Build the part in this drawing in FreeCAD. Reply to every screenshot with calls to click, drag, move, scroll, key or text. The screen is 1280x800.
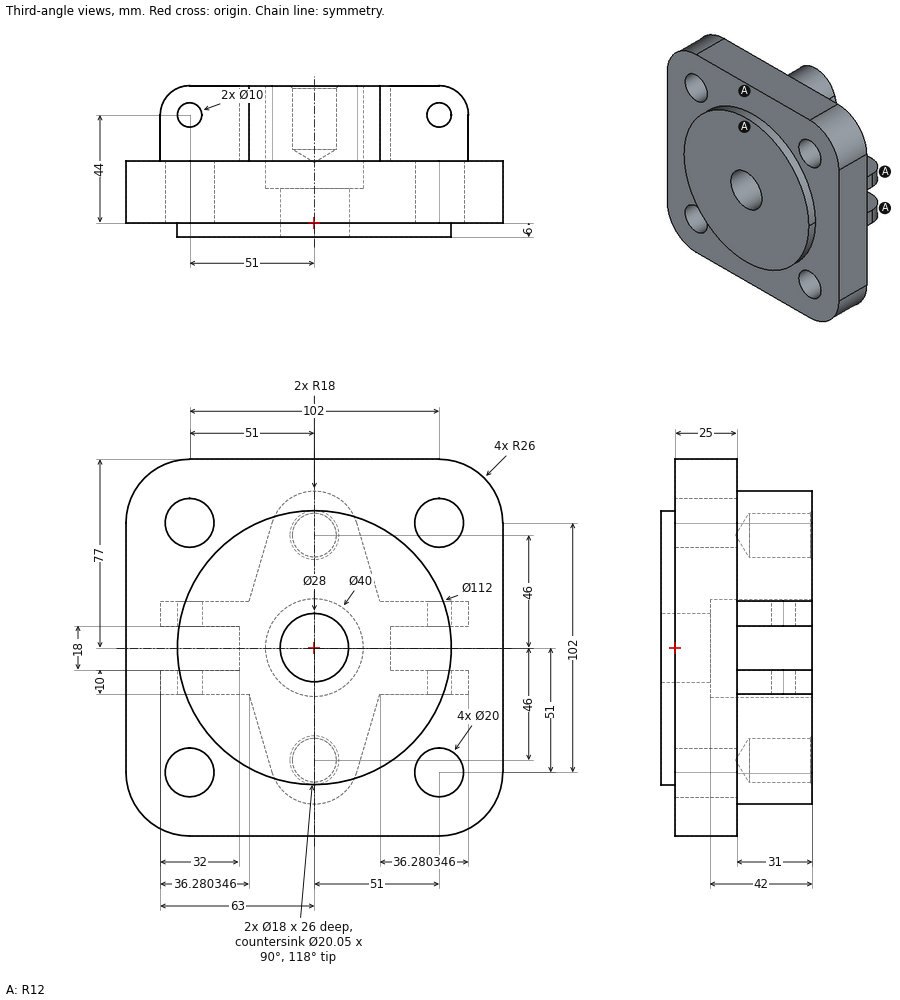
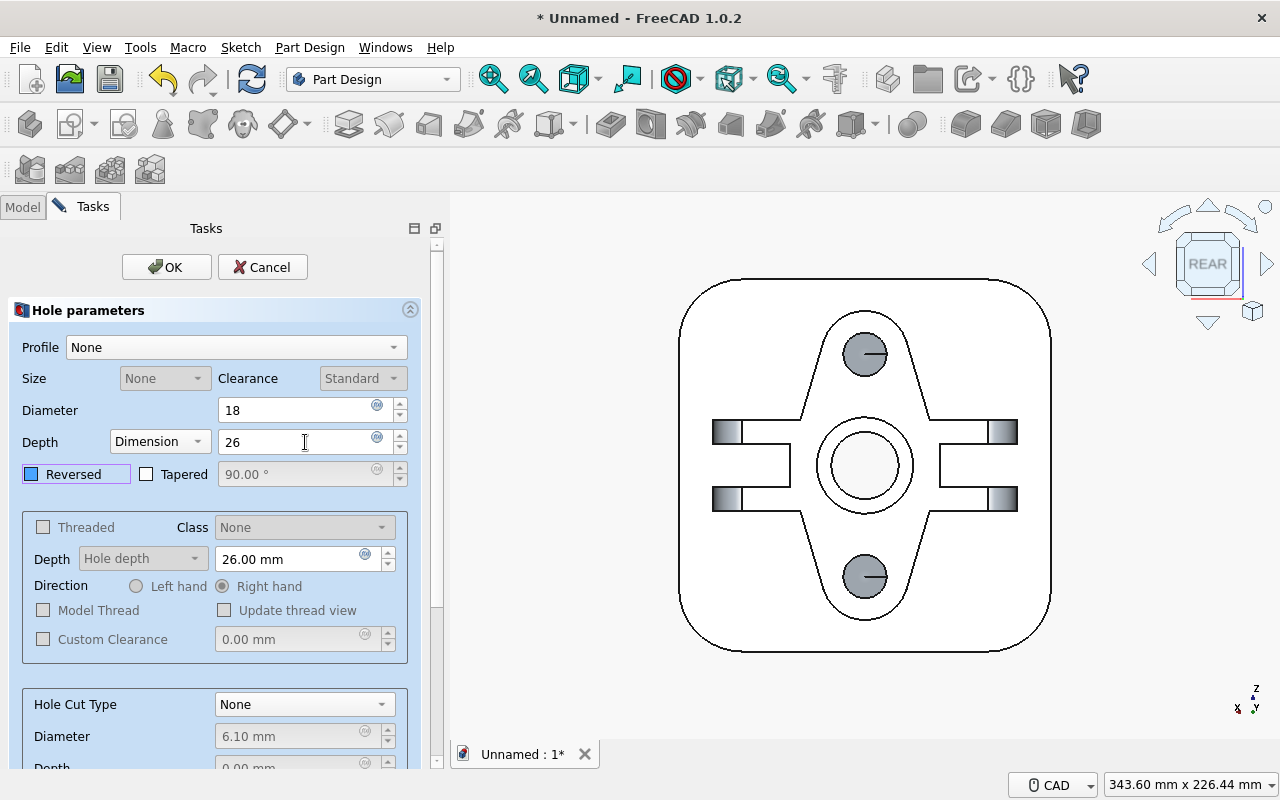
click(306, 704)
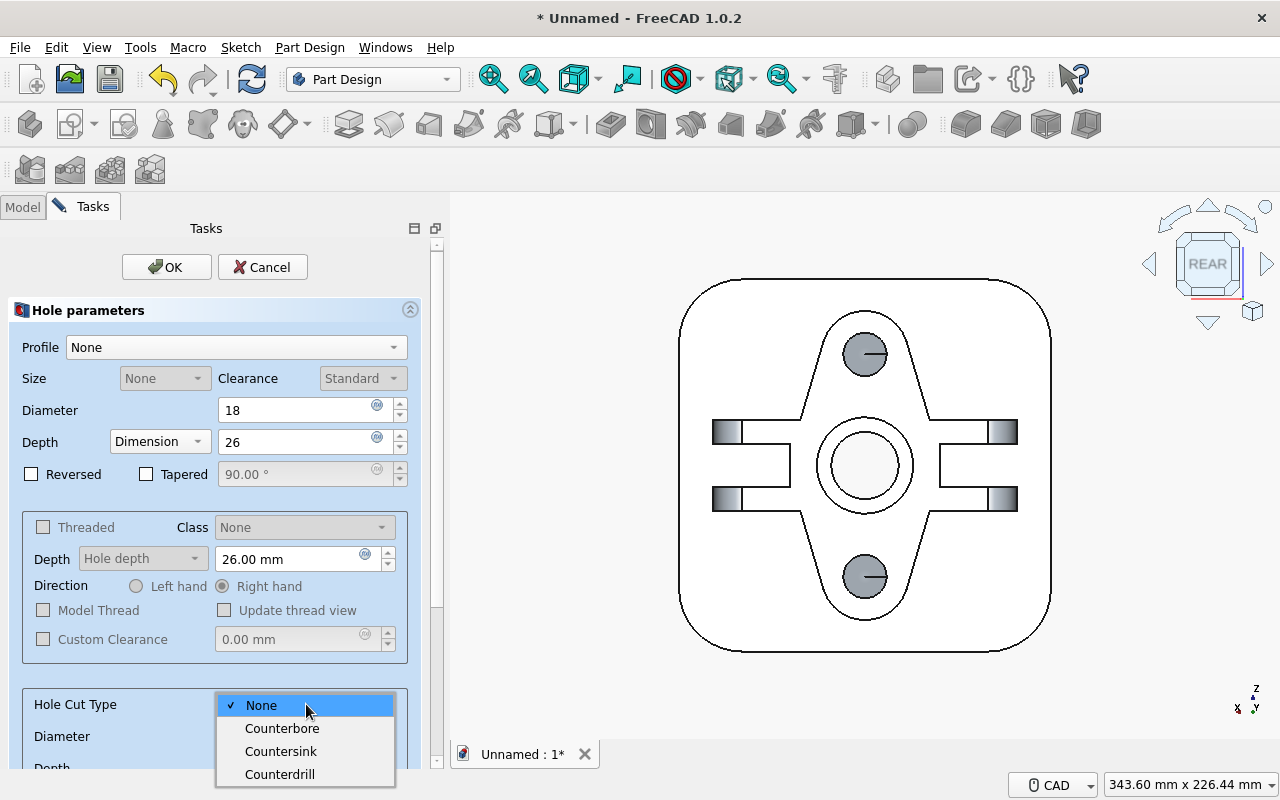
click(304, 752)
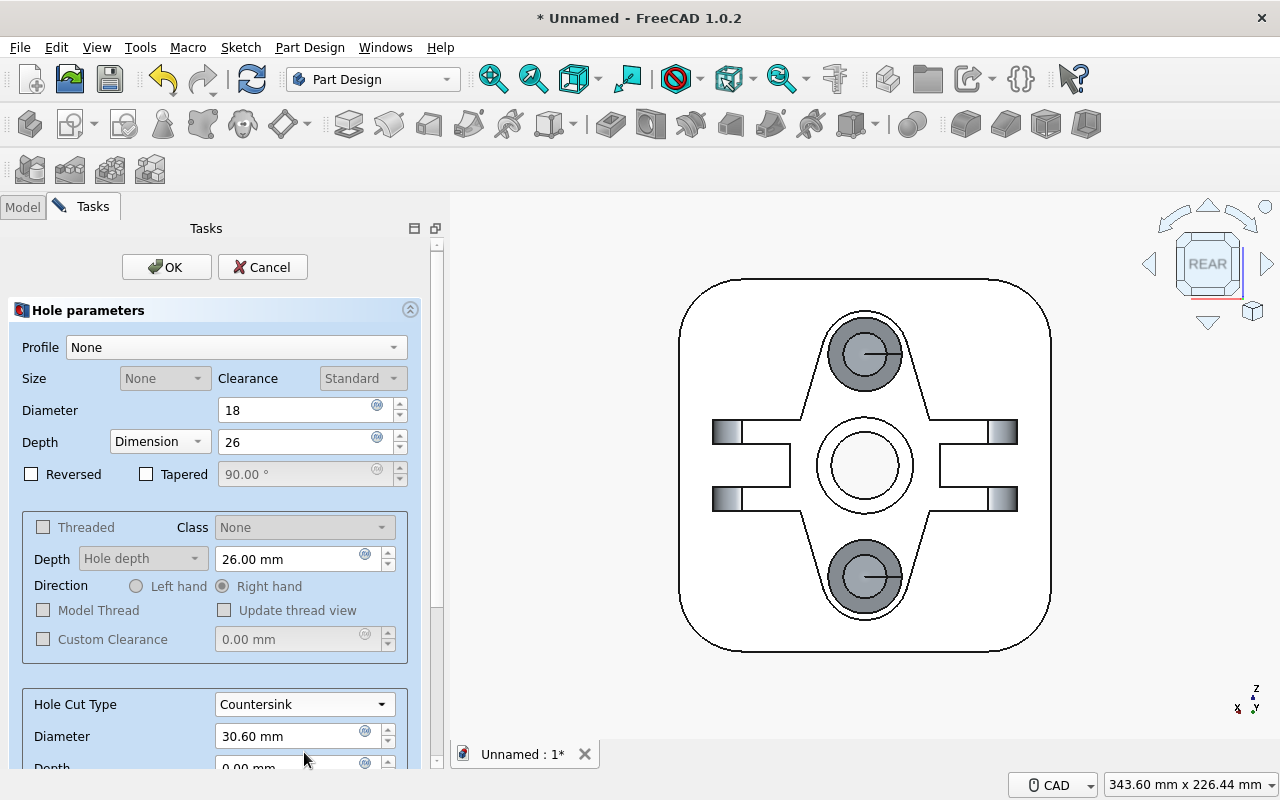
triple_click(298, 736)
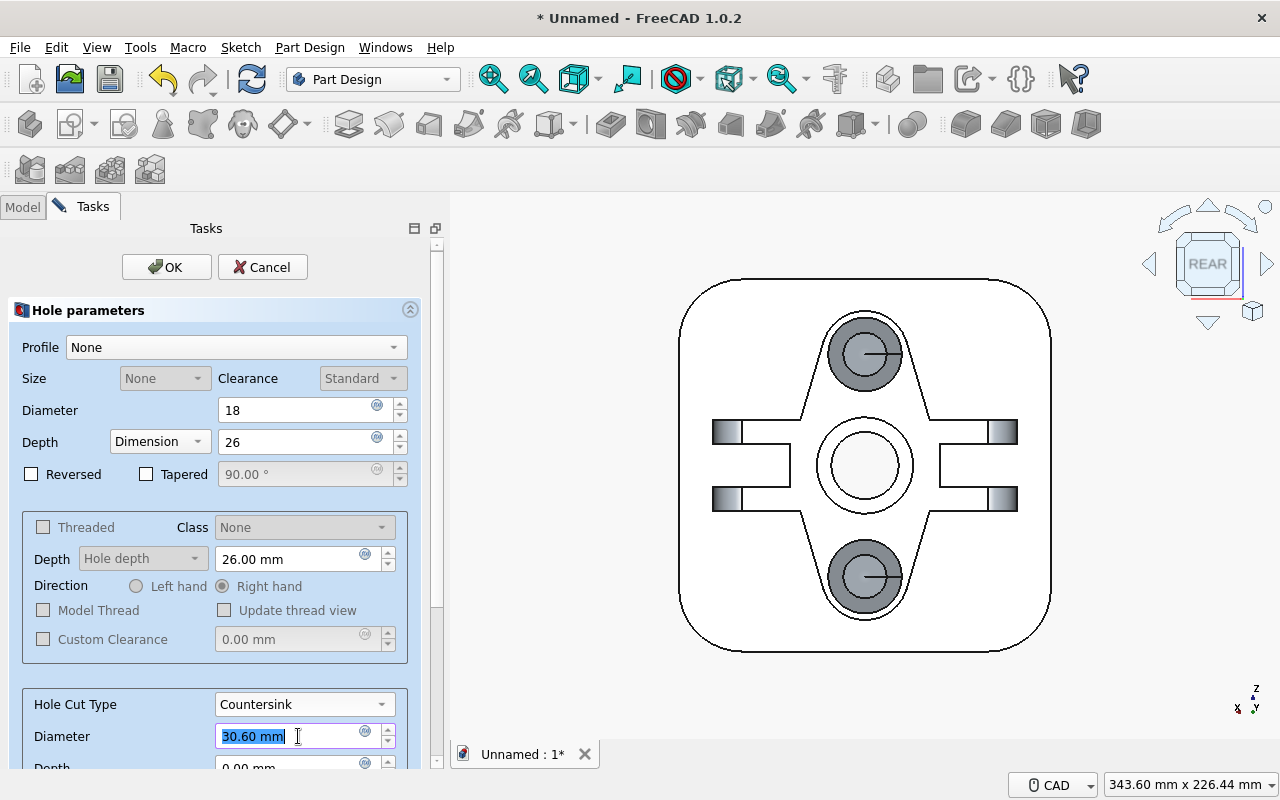
text(20.05)
key(Tab)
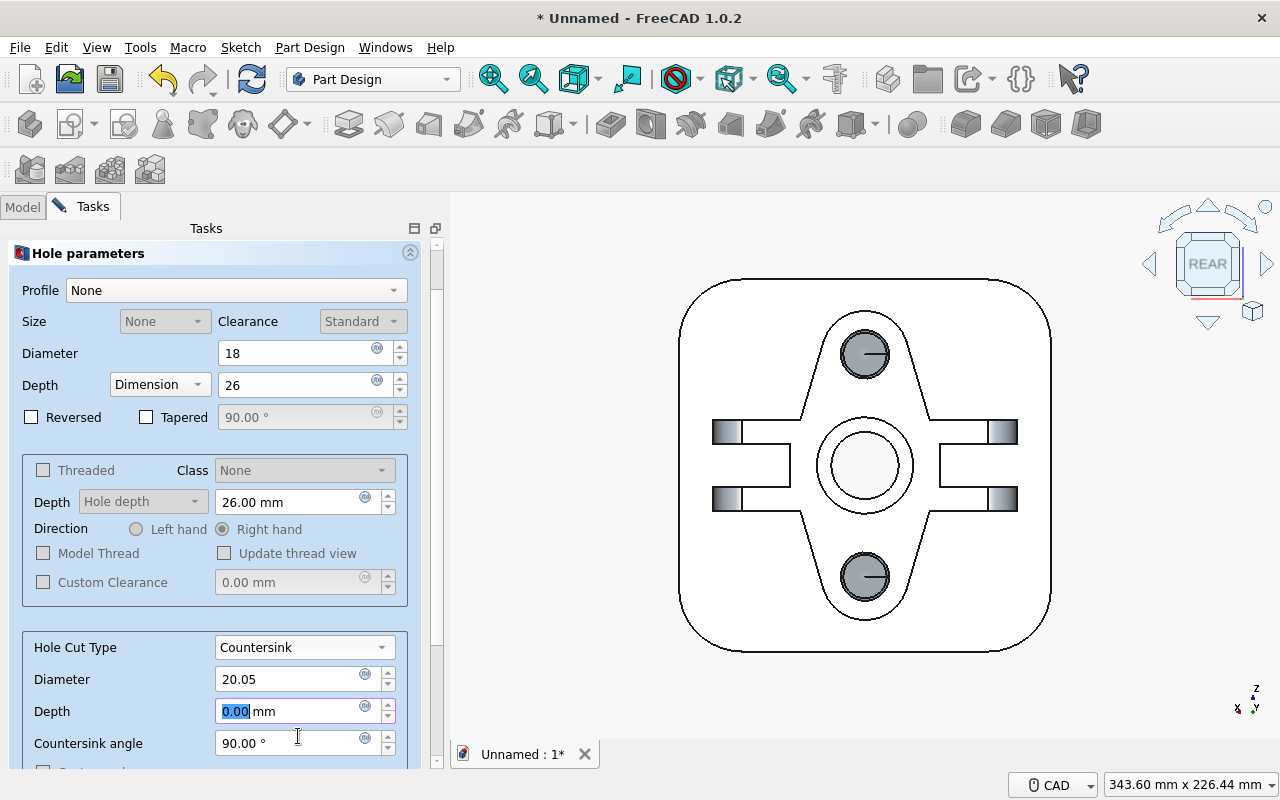
scroll(437, 503, up, 2)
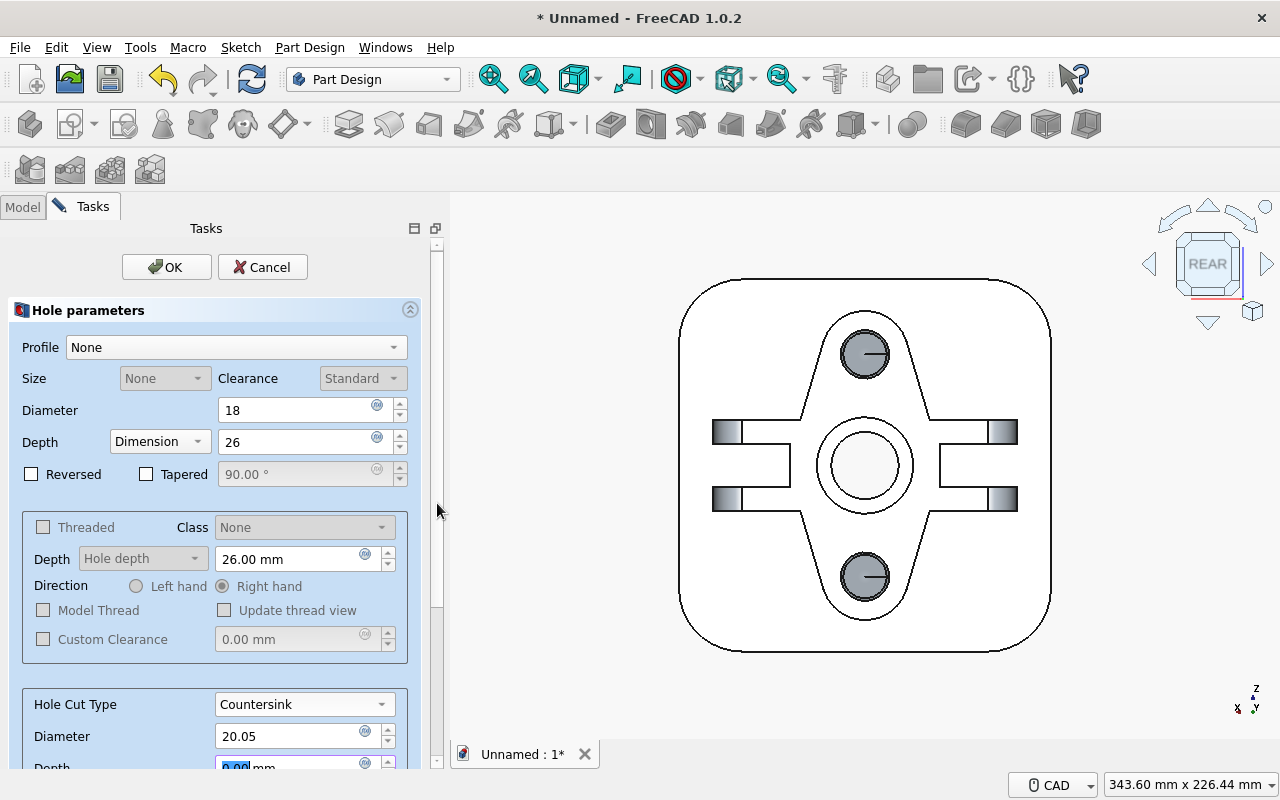
click(167, 267)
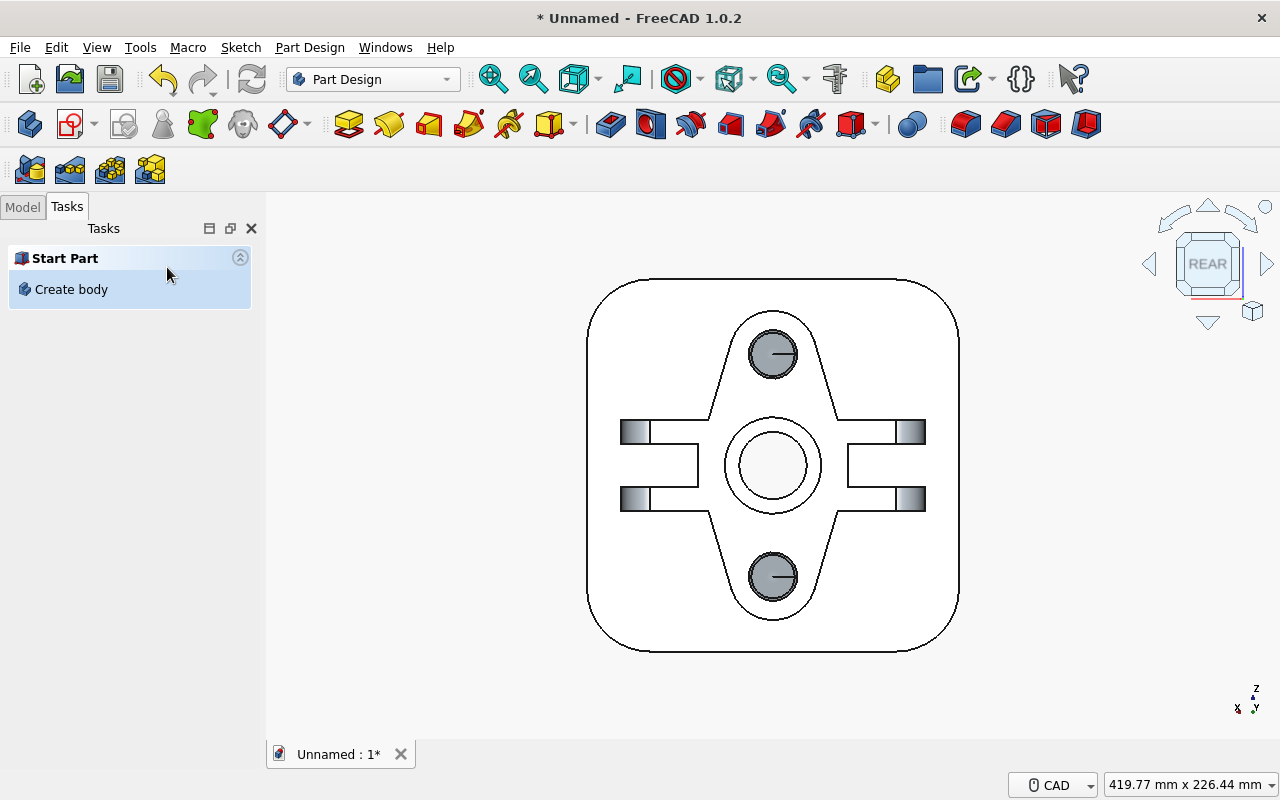
click(667, 571)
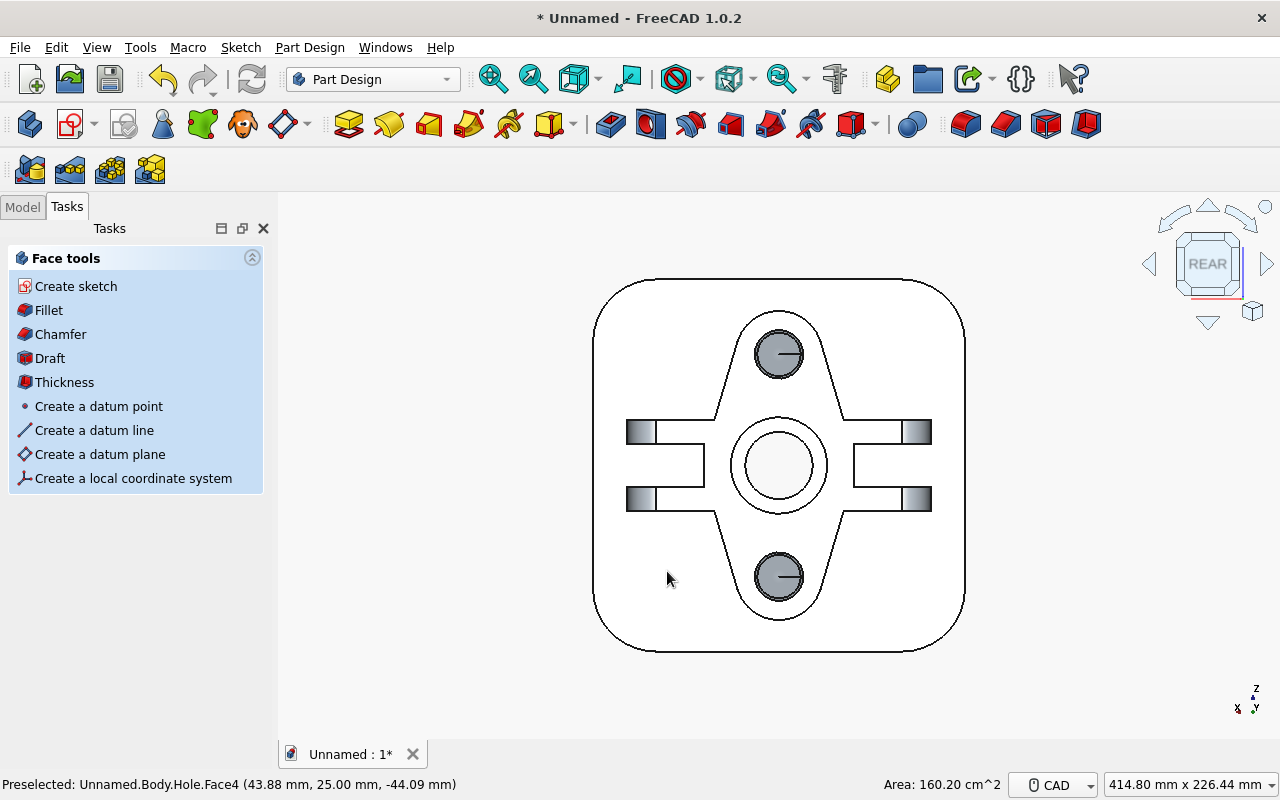
click(70, 124)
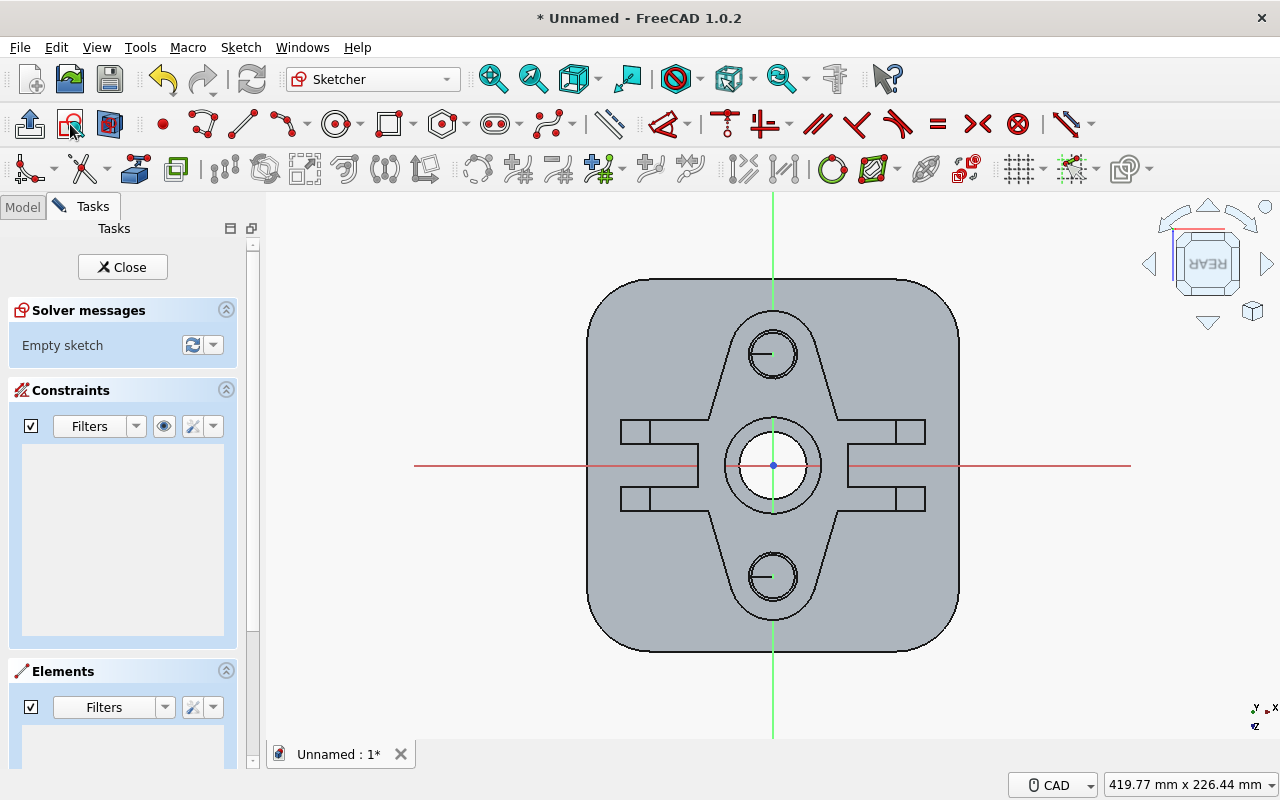
key(g)
key(c)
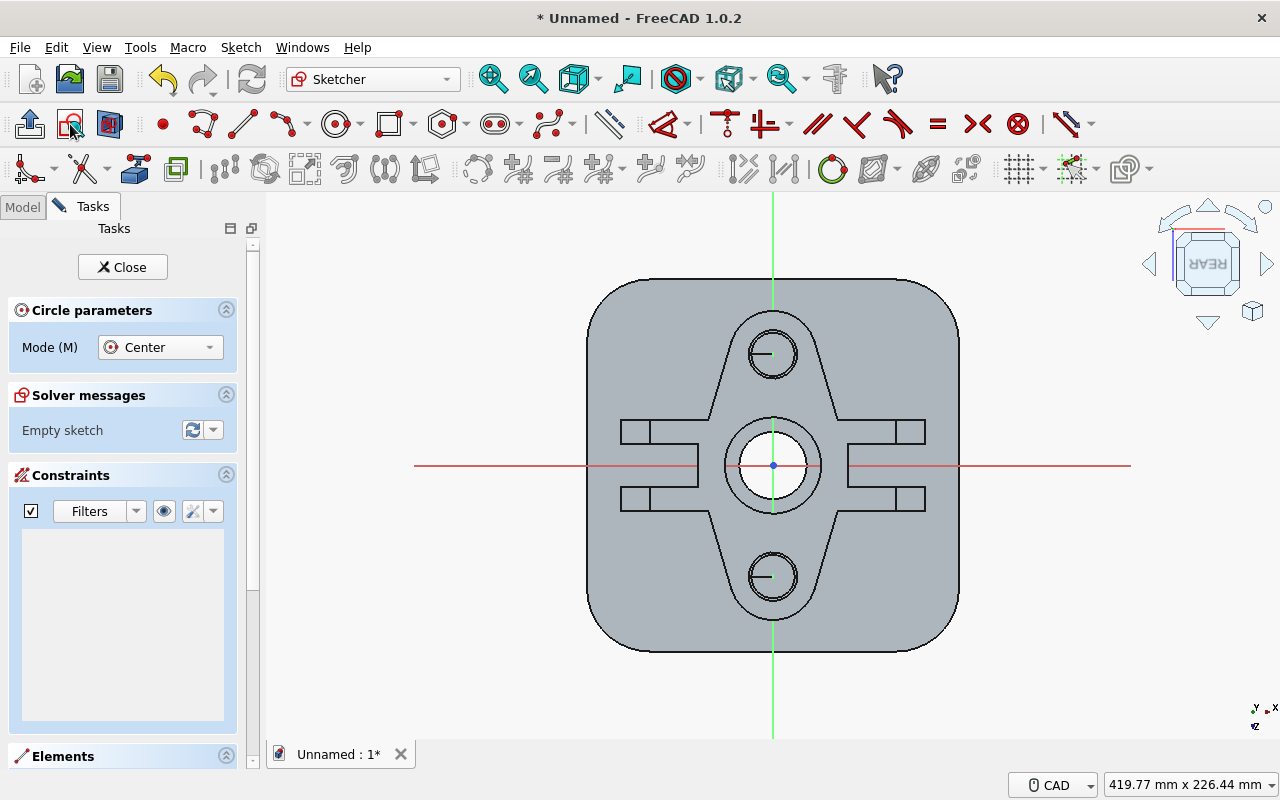
click(896, 342)
click(913, 325)